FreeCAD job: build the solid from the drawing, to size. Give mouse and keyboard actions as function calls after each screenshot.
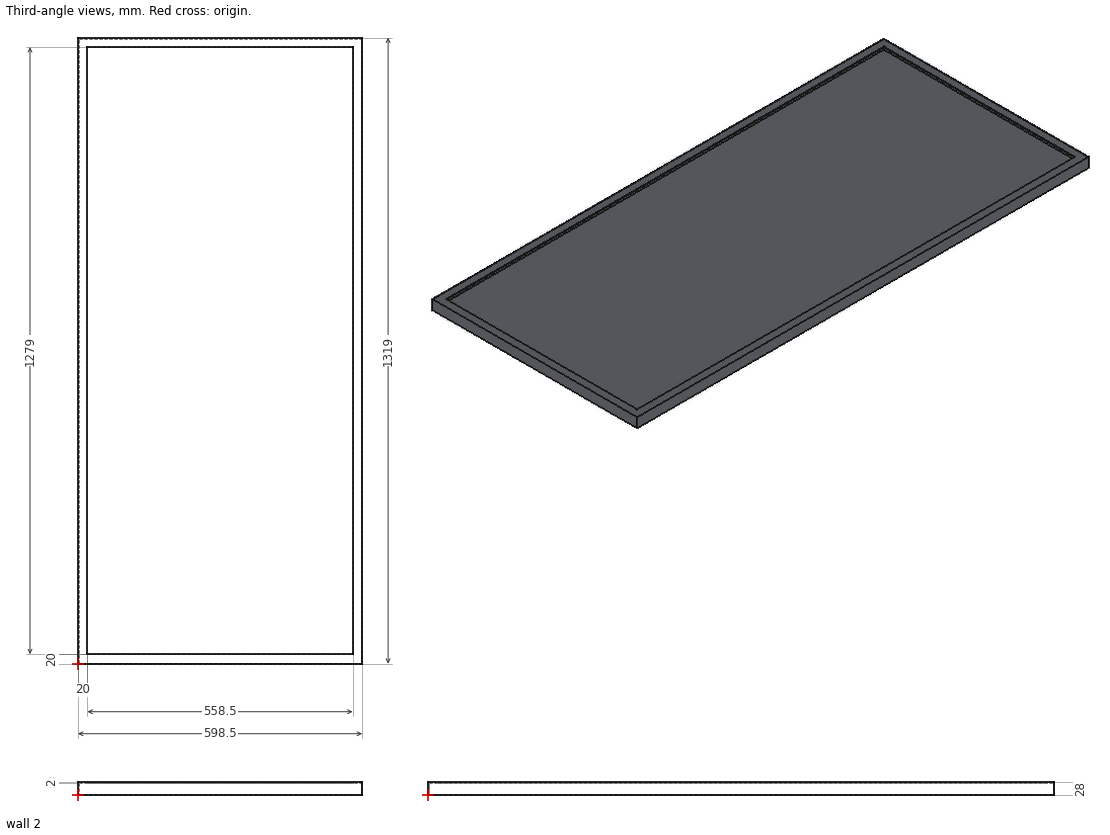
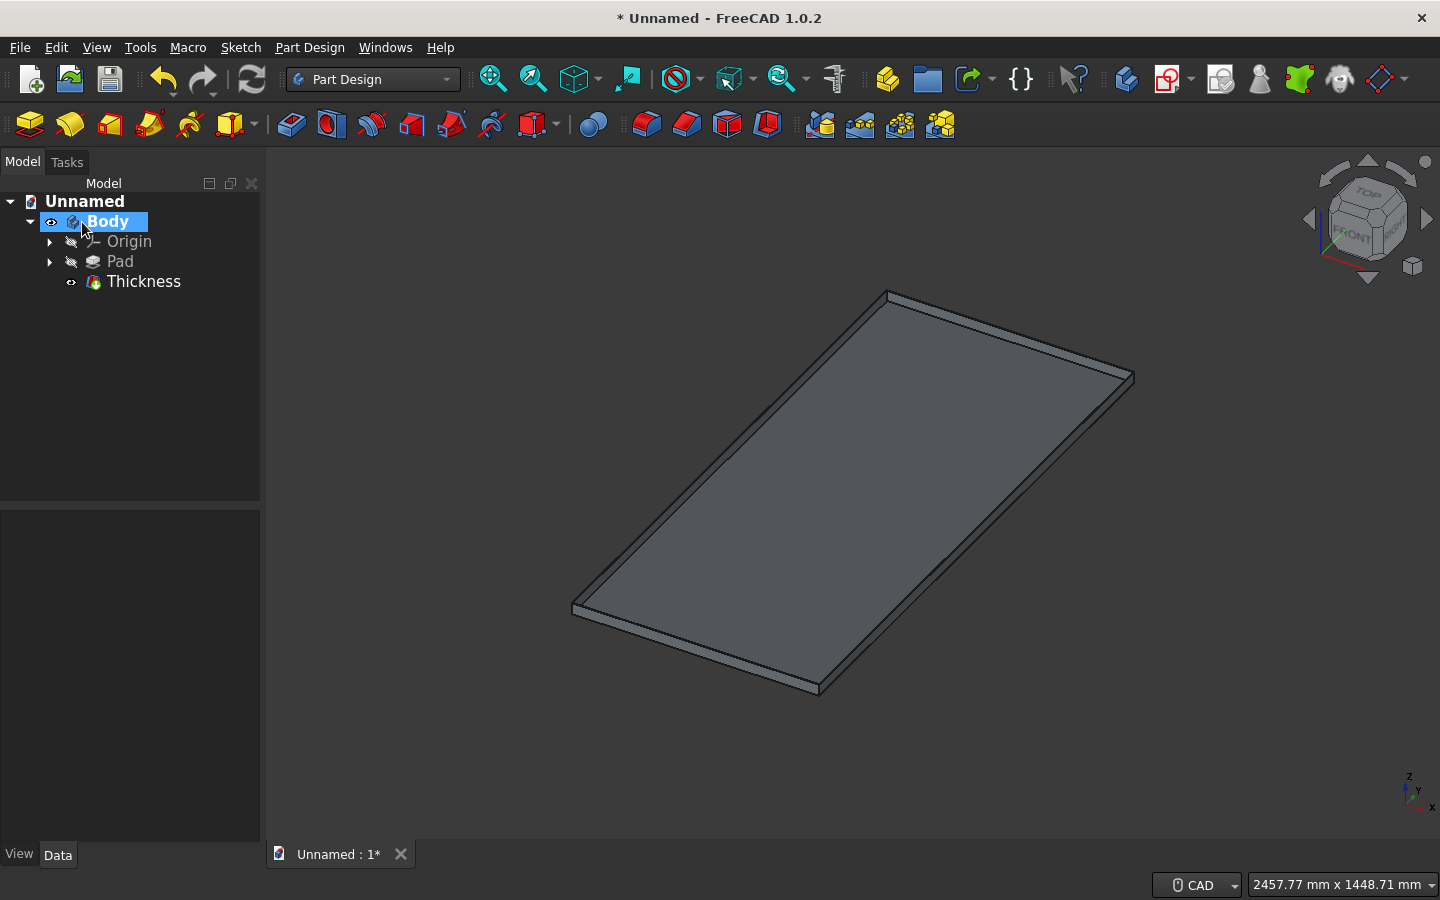
scroll(1051, 344, up, 15)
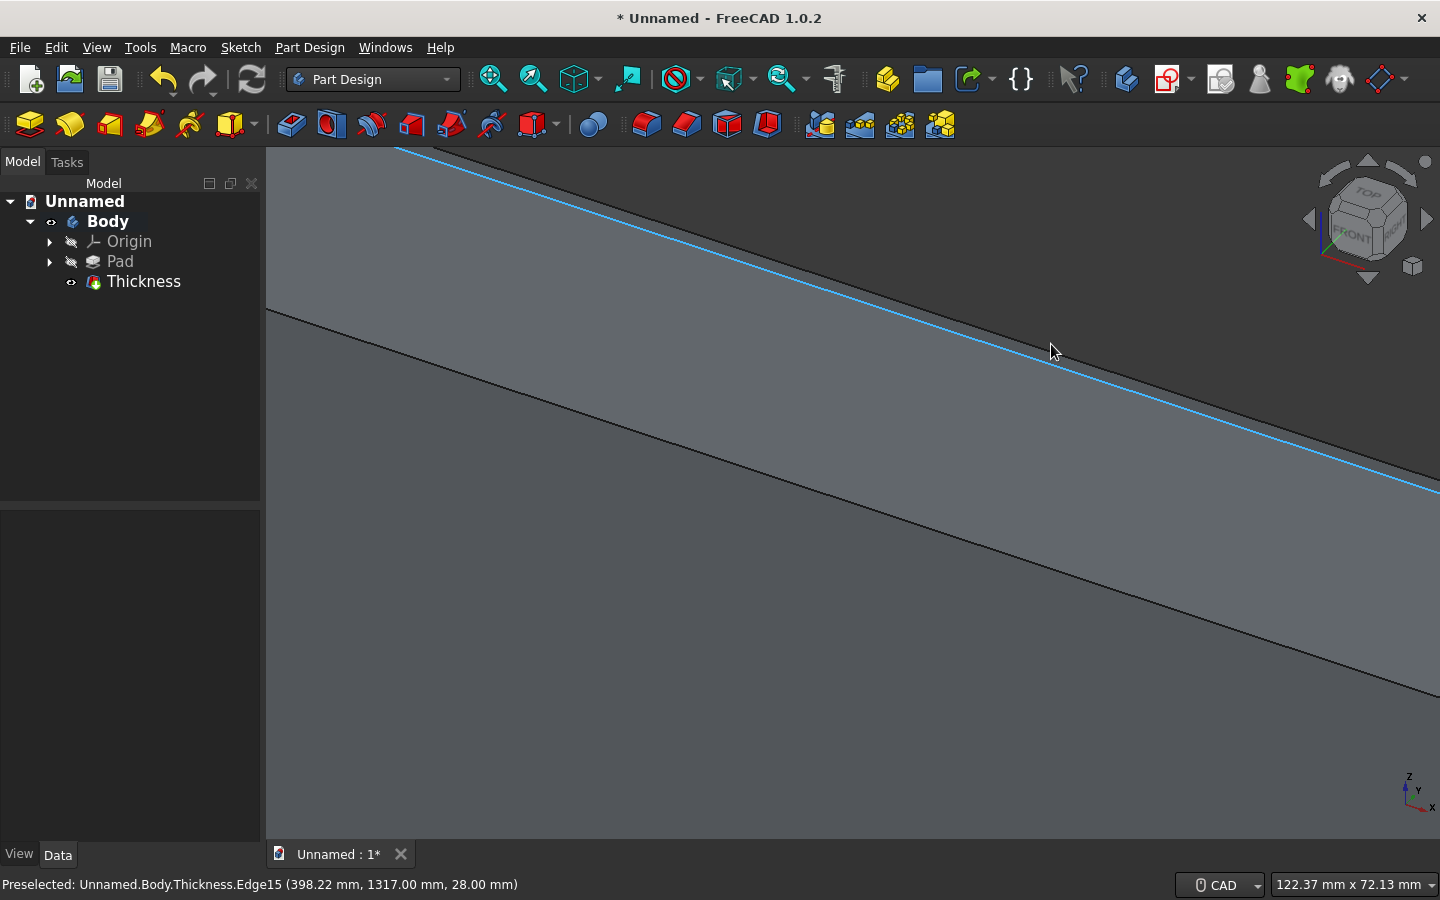
scroll(1047, 358, up, 4)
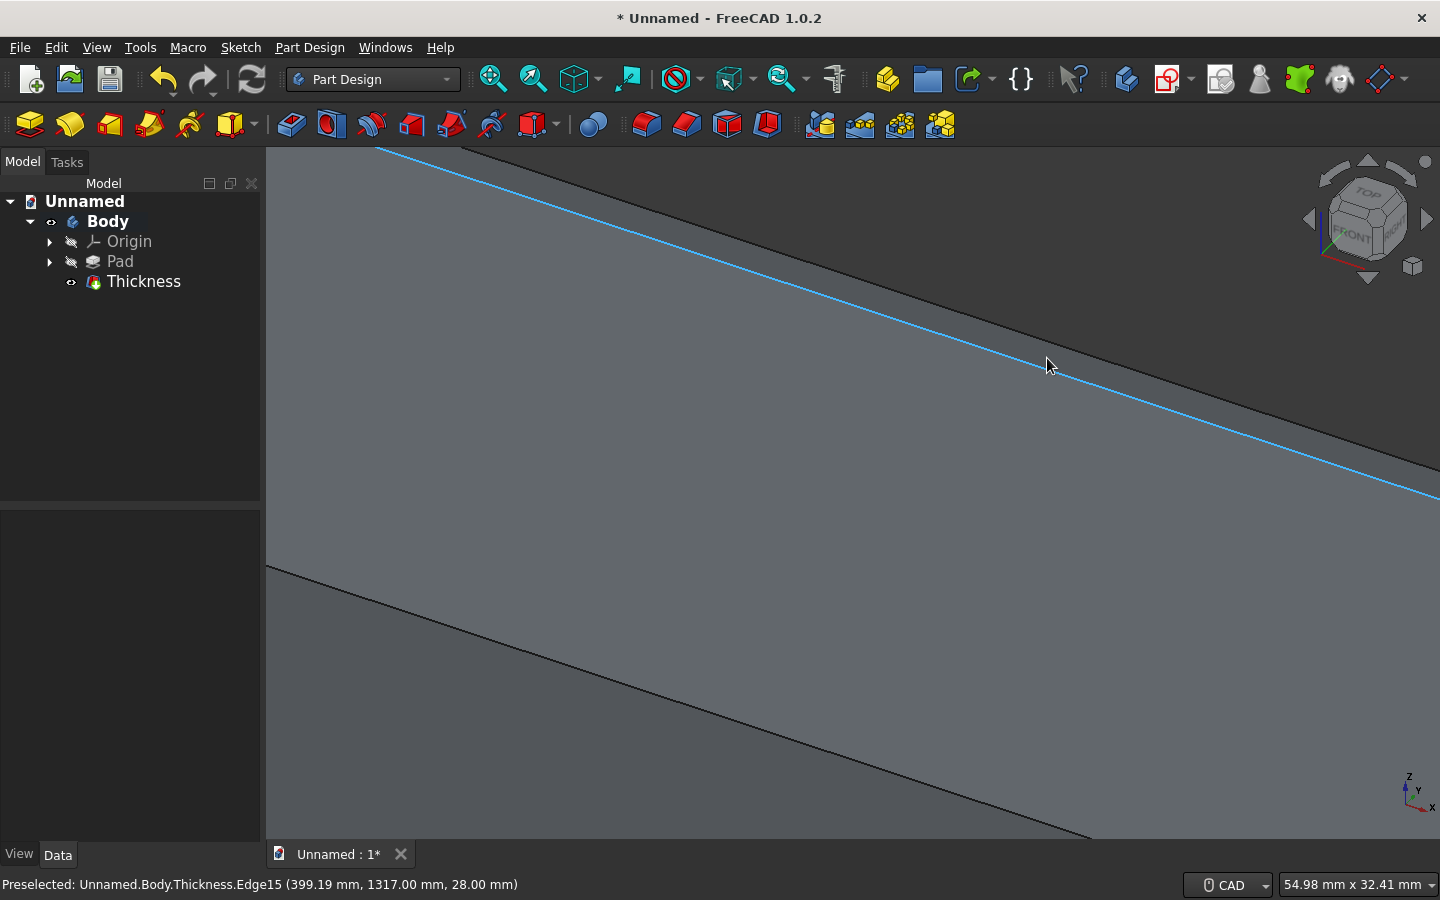
click(1047, 359)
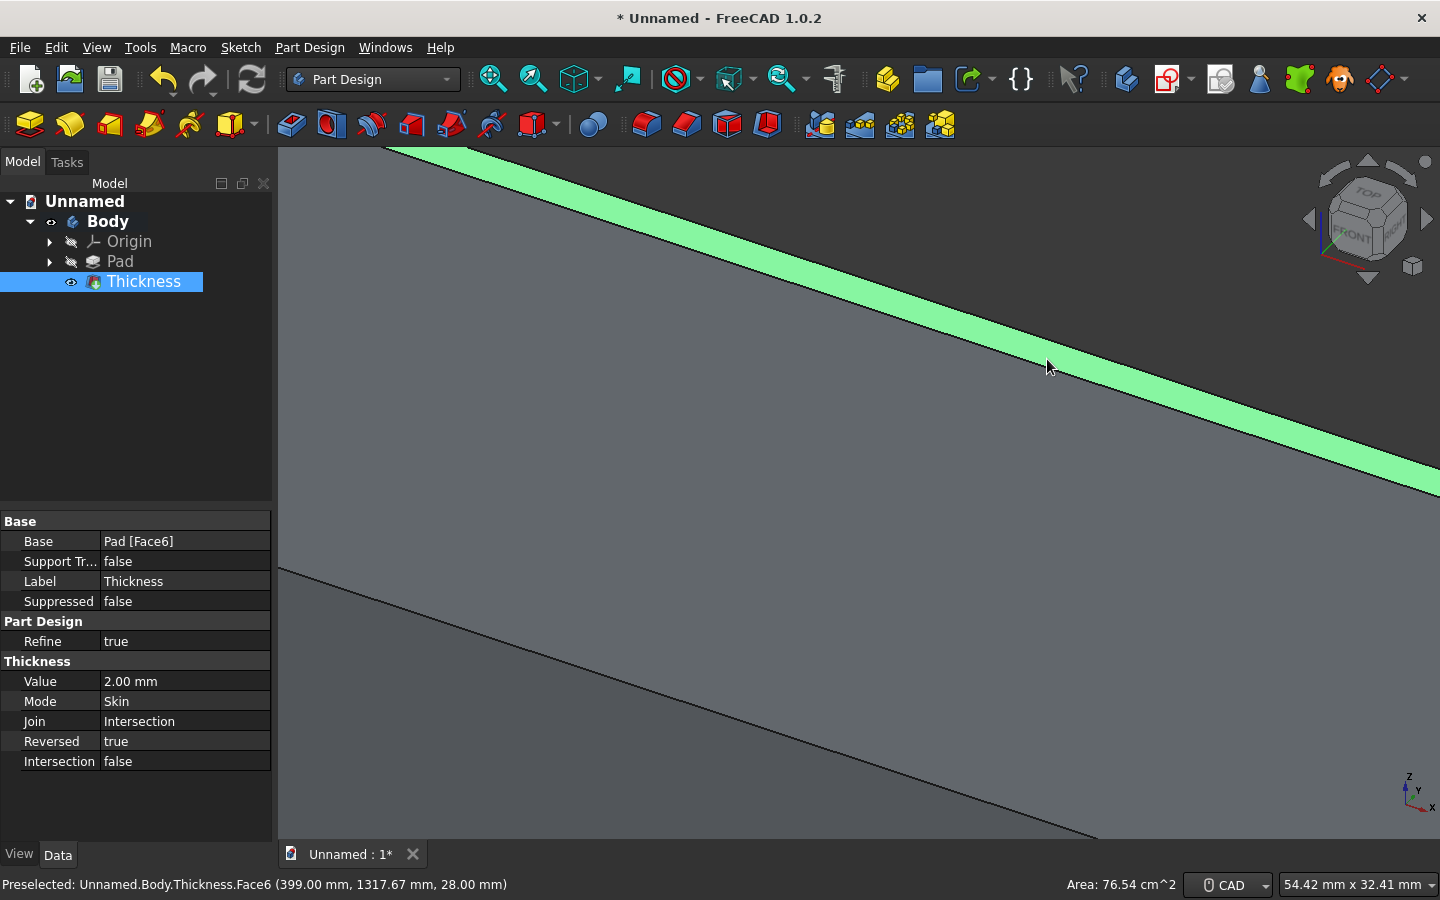
click(1168, 80)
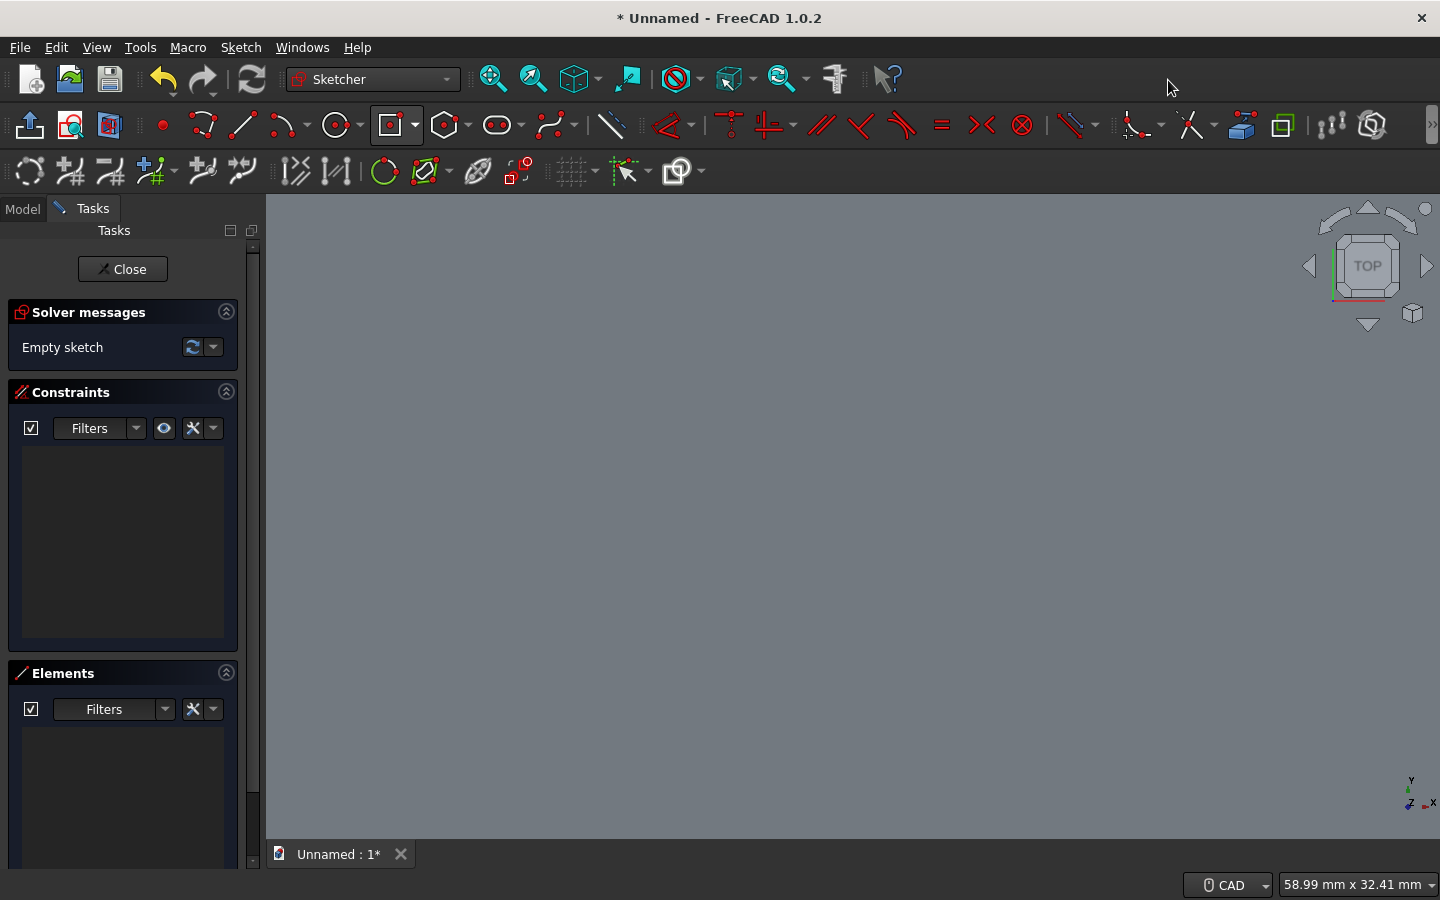
scroll(784, 516, down, 15)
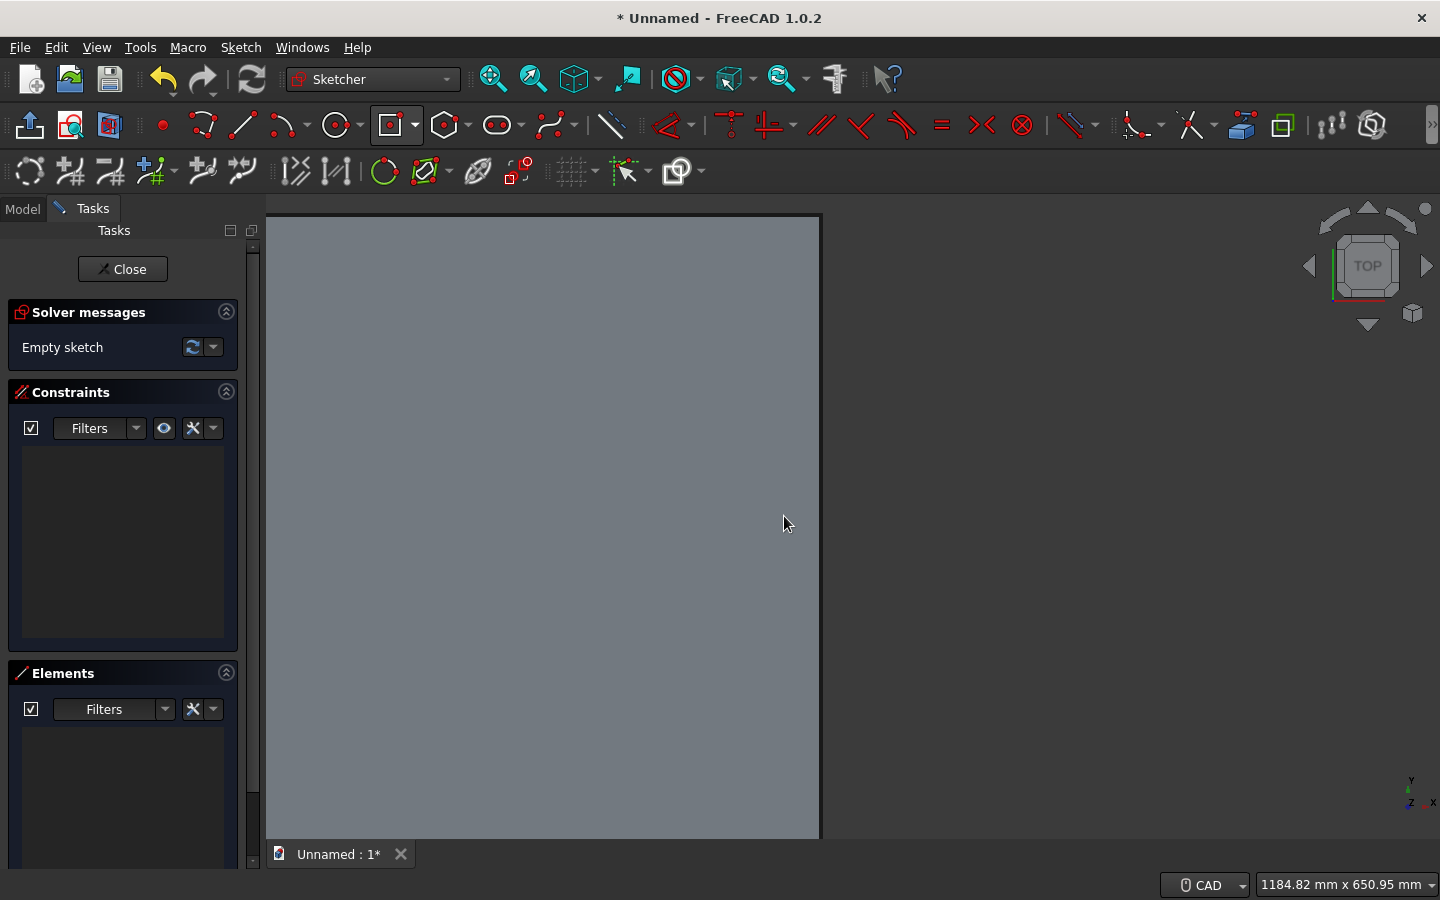
scroll(896, 365, down, 6)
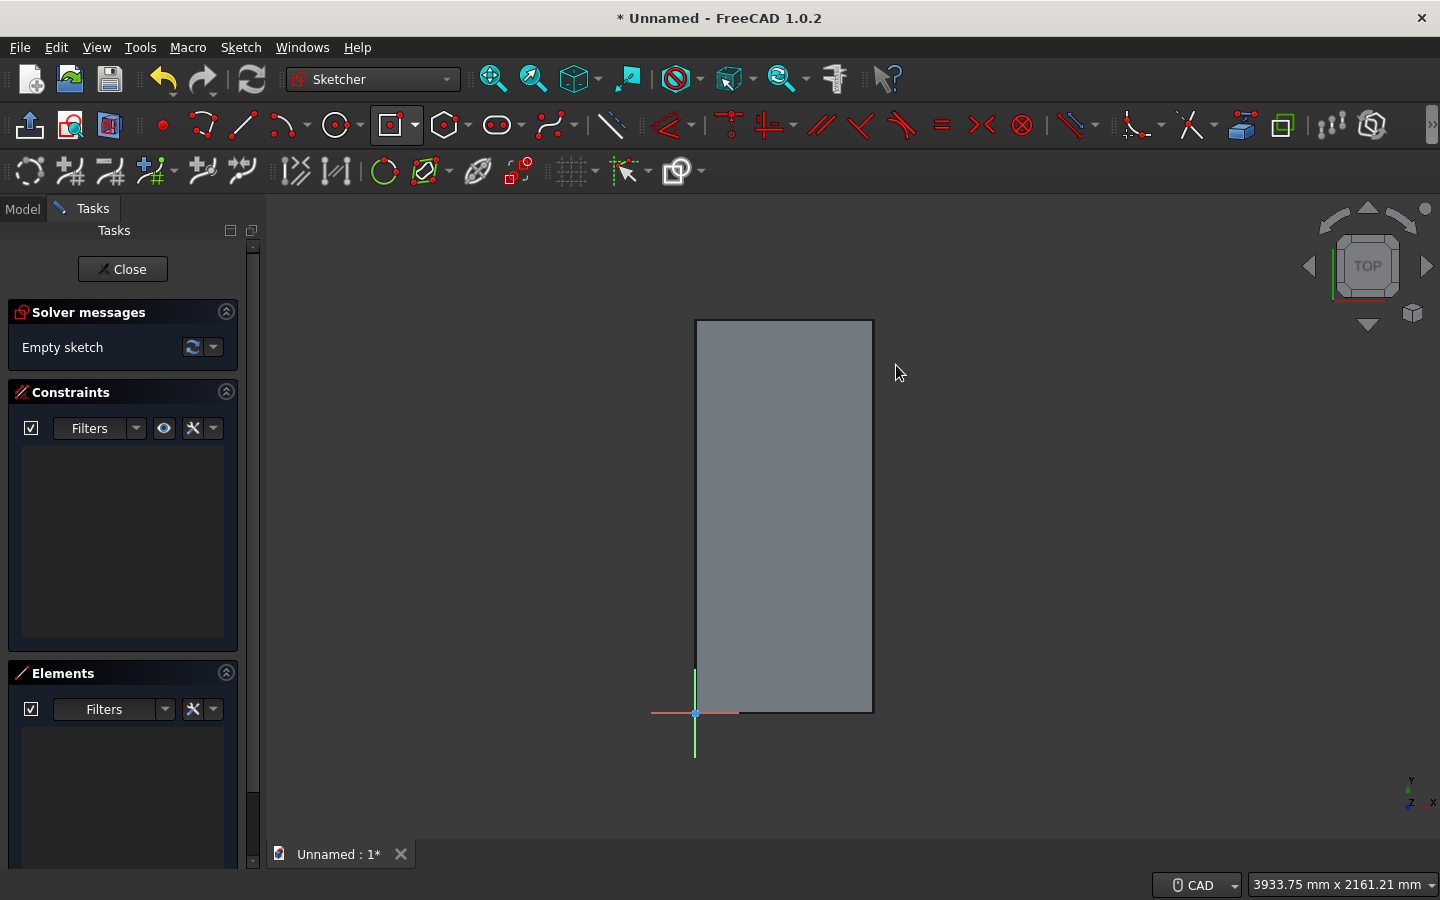
click(418, 126)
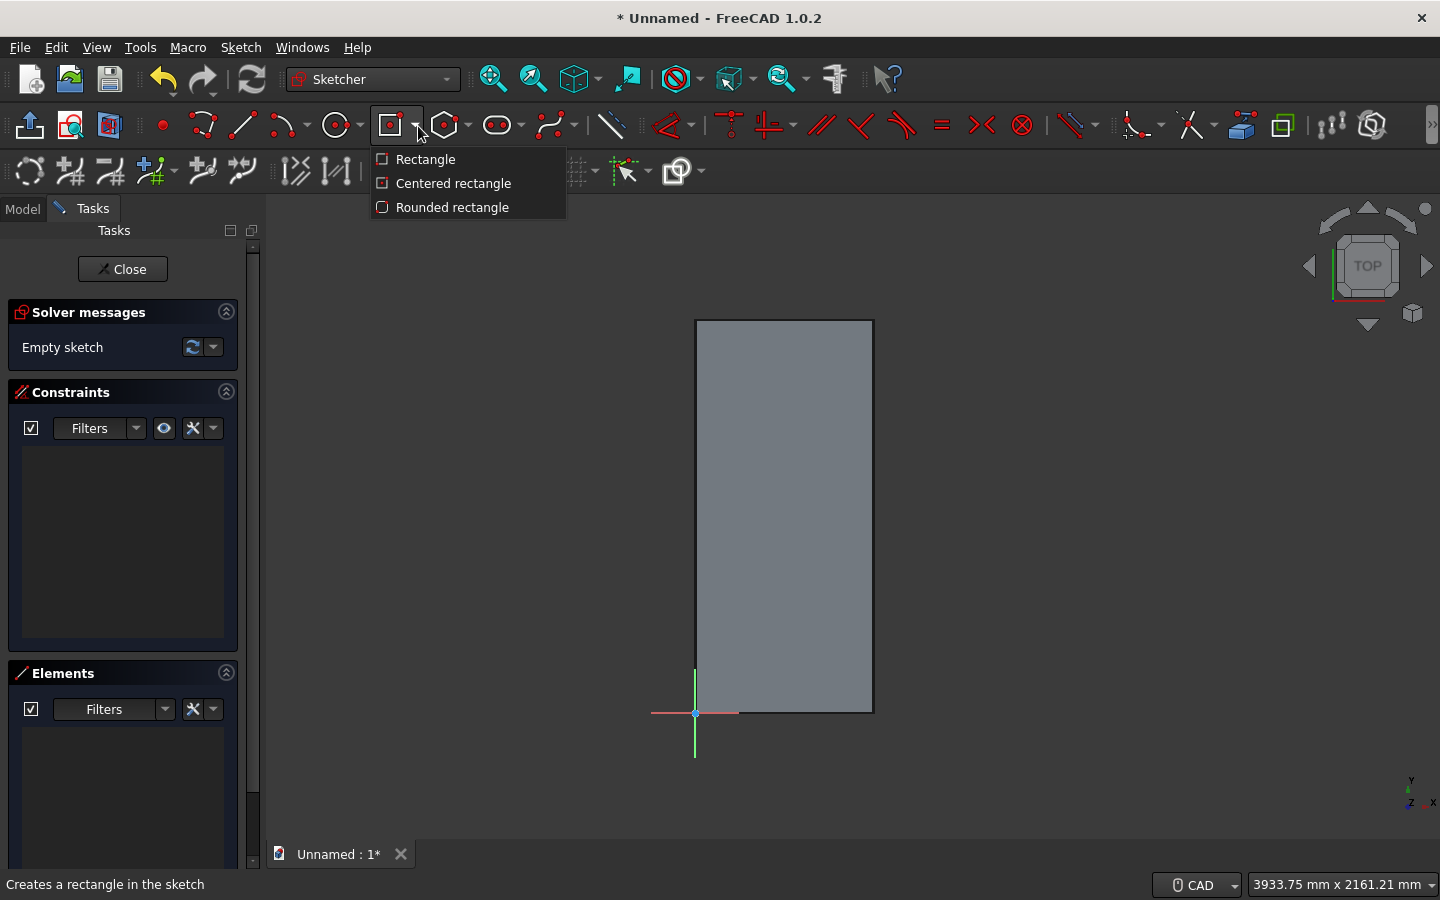
click(468, 159)